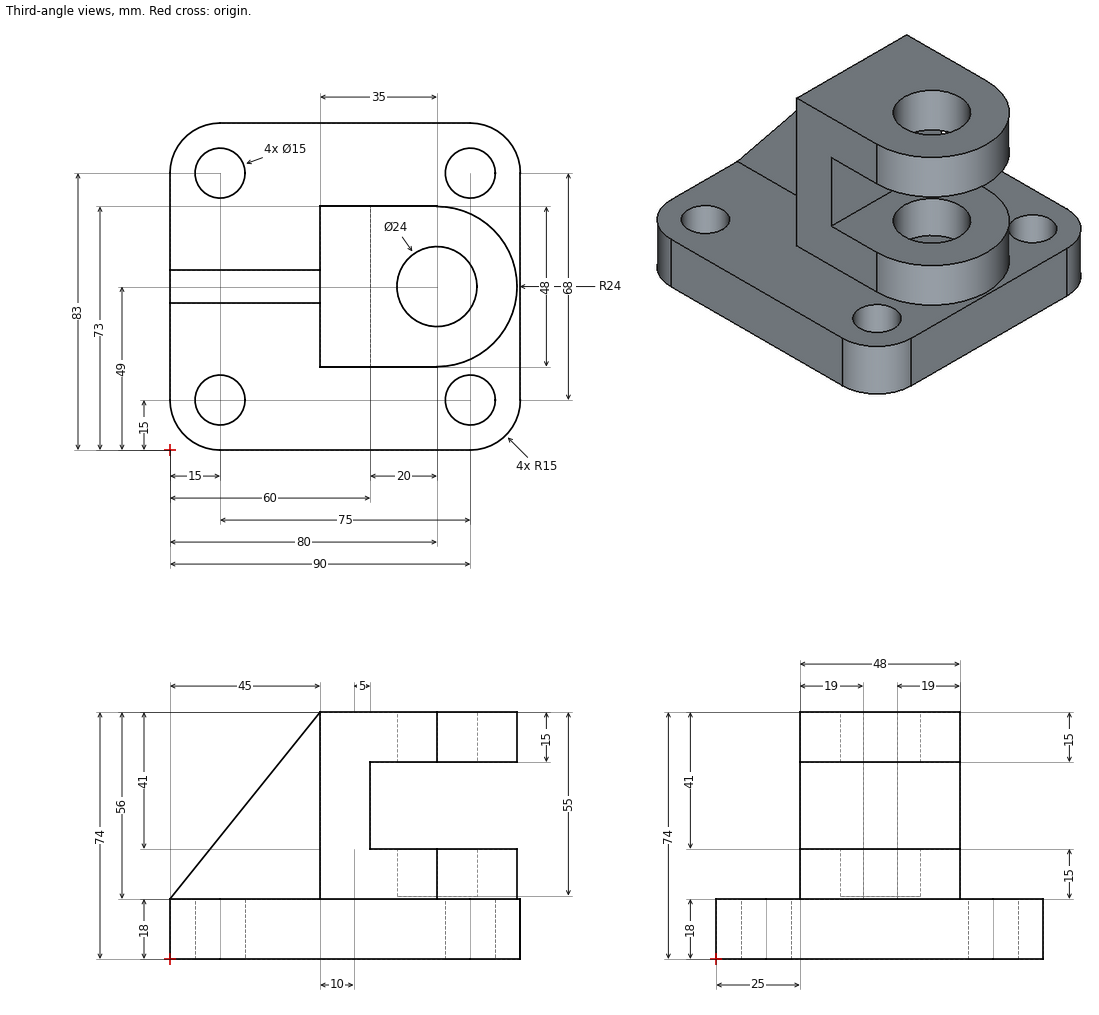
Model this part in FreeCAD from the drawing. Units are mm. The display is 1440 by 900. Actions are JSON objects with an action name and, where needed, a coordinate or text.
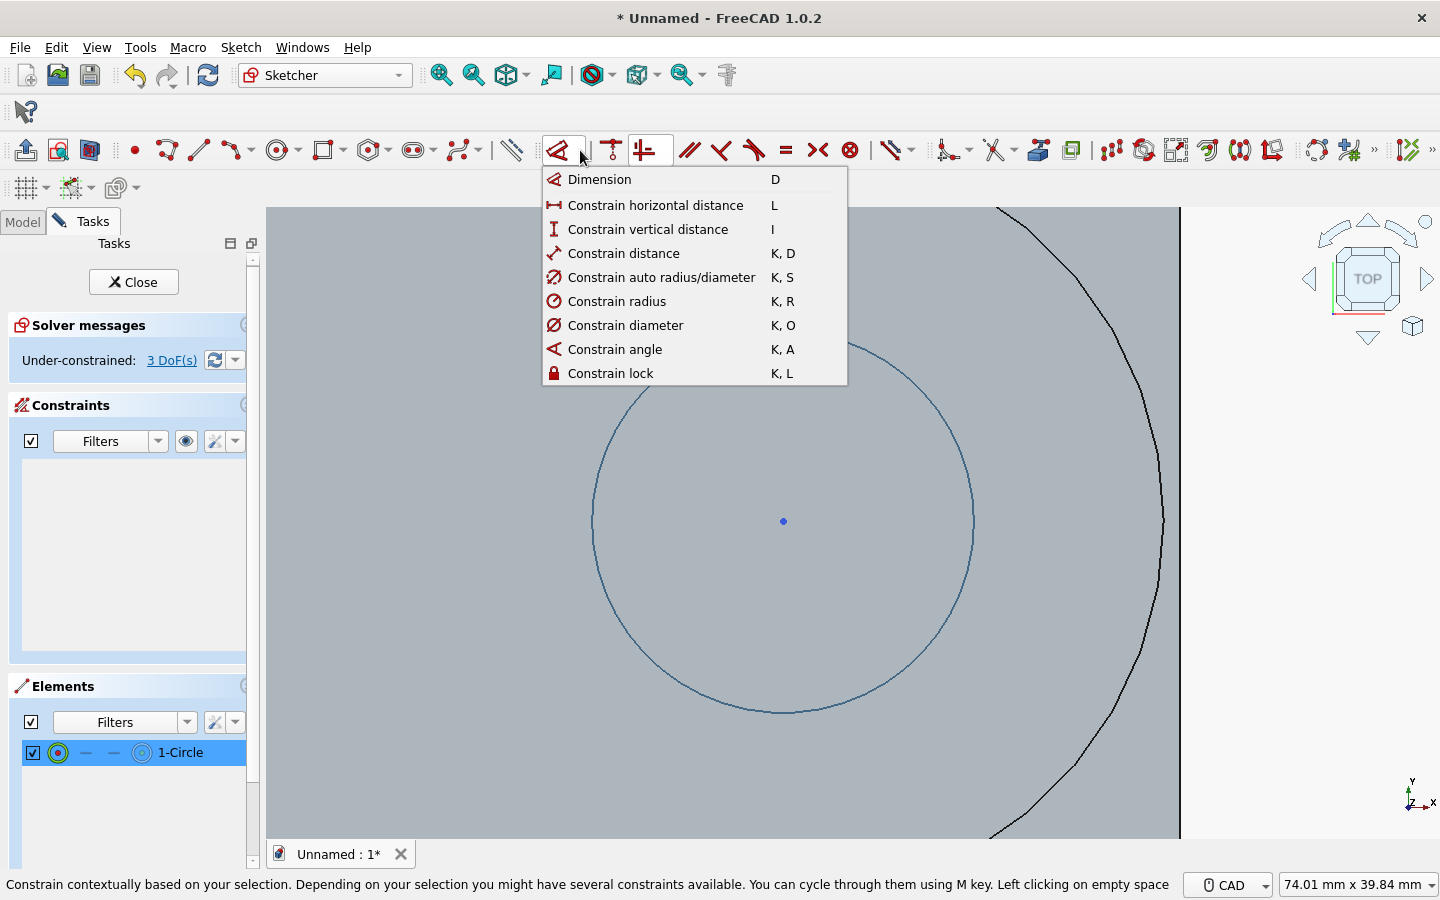
{"action": "left_click", "coordinate": [695, 325]}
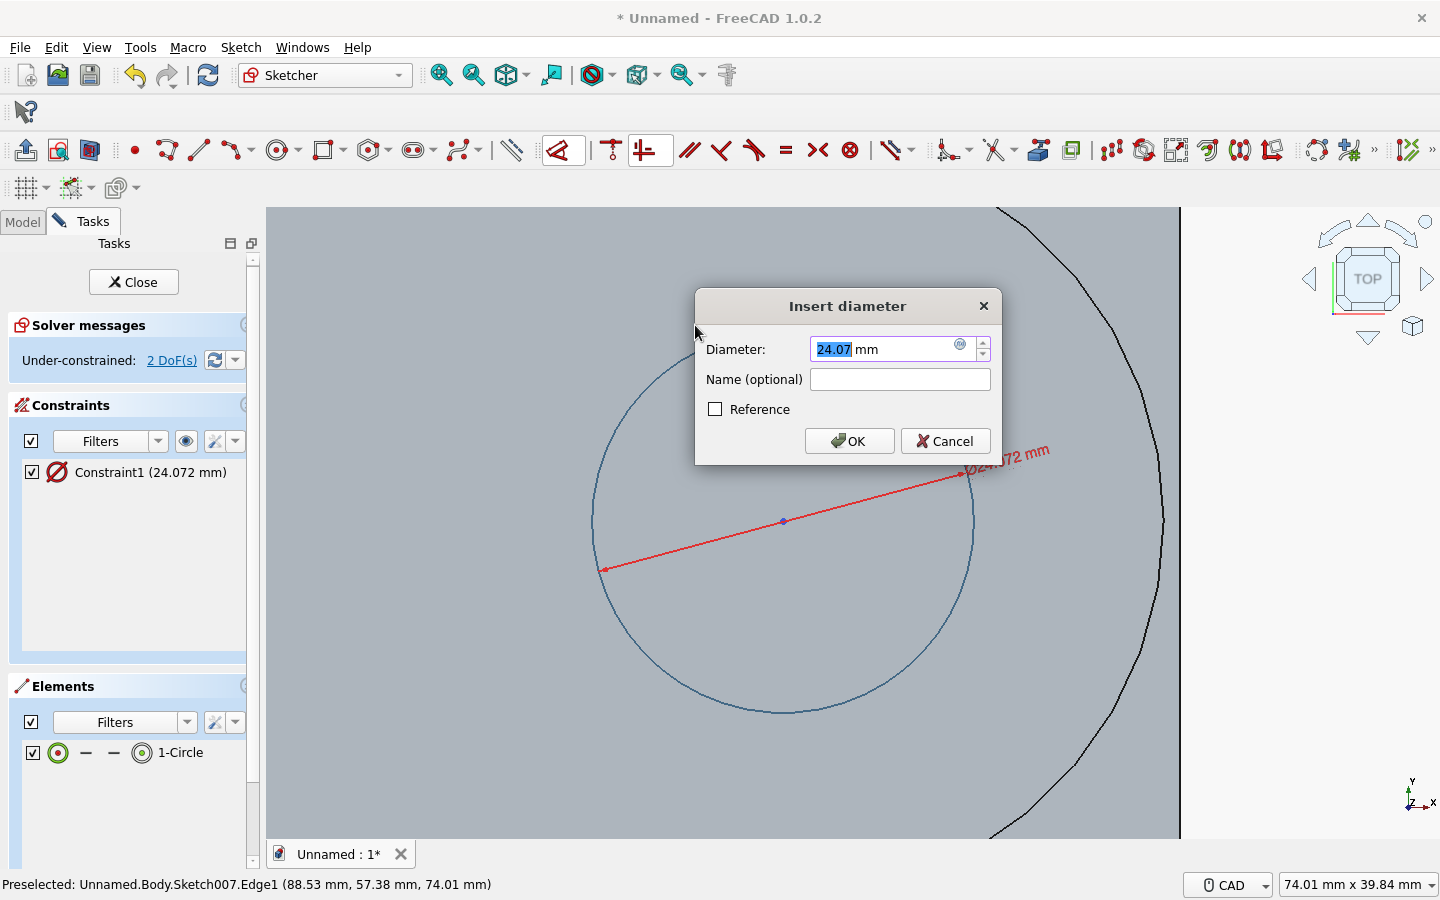
{"action": "type", "text": "24"}
{"action": "key", "text": "Return"}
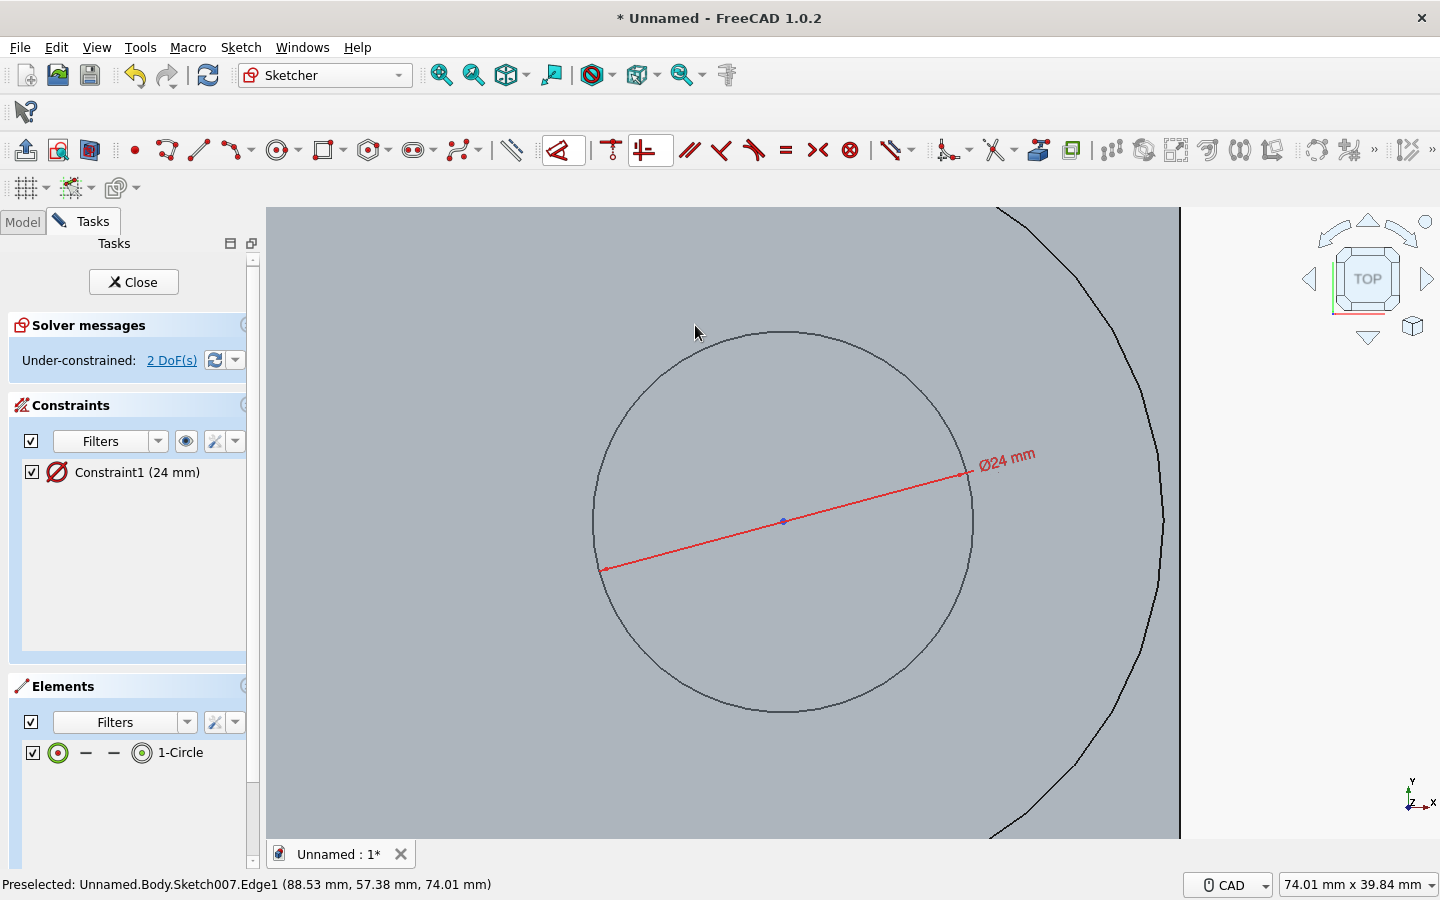
{"action": "left_click", "coordinate": [783, 522]}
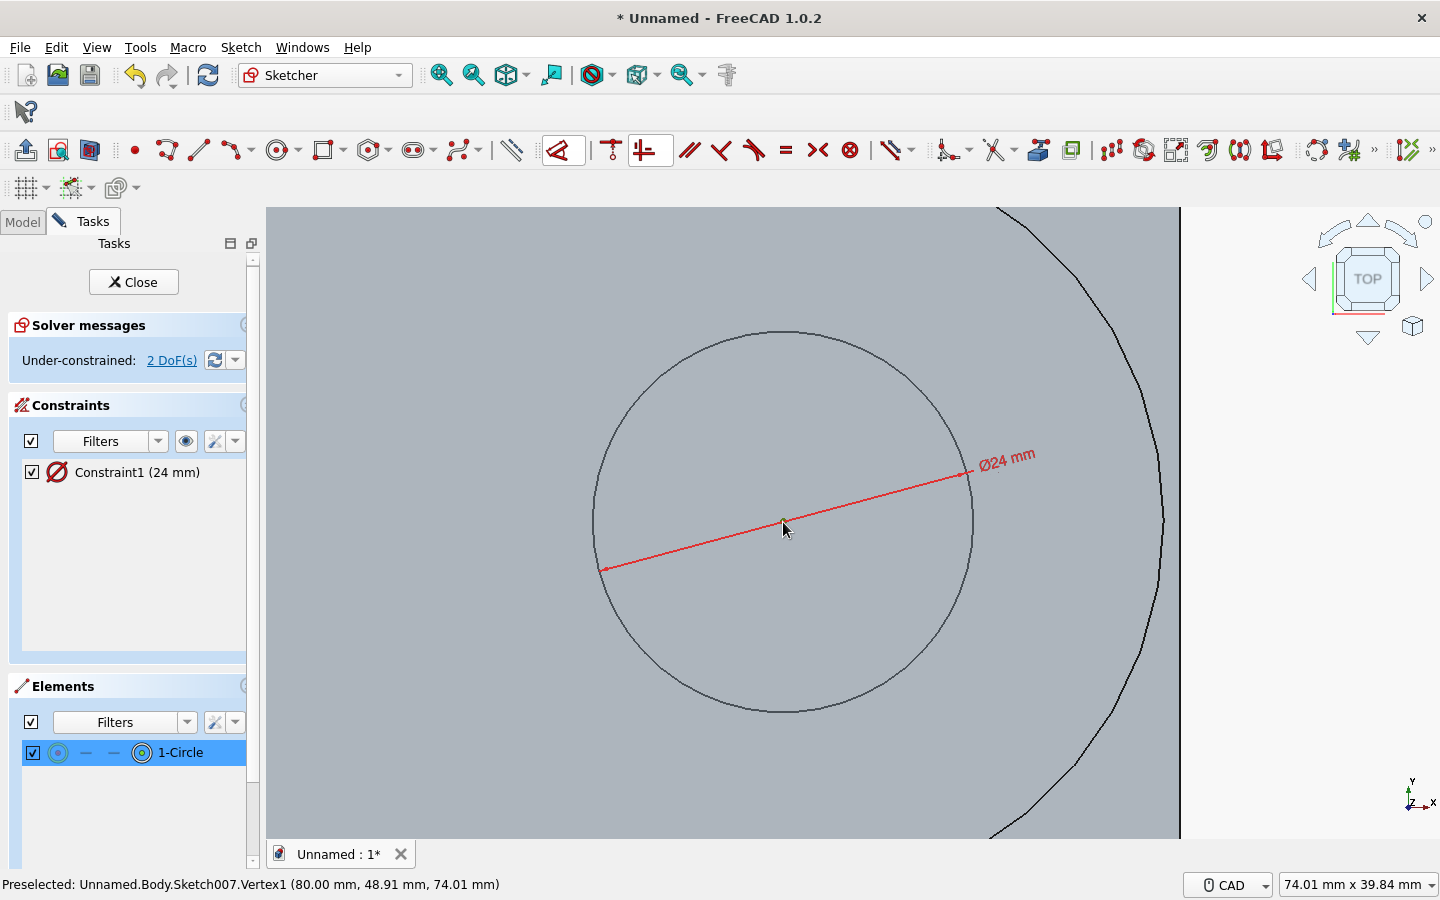
{"action": "left_click", "coordinate": [580, 150]}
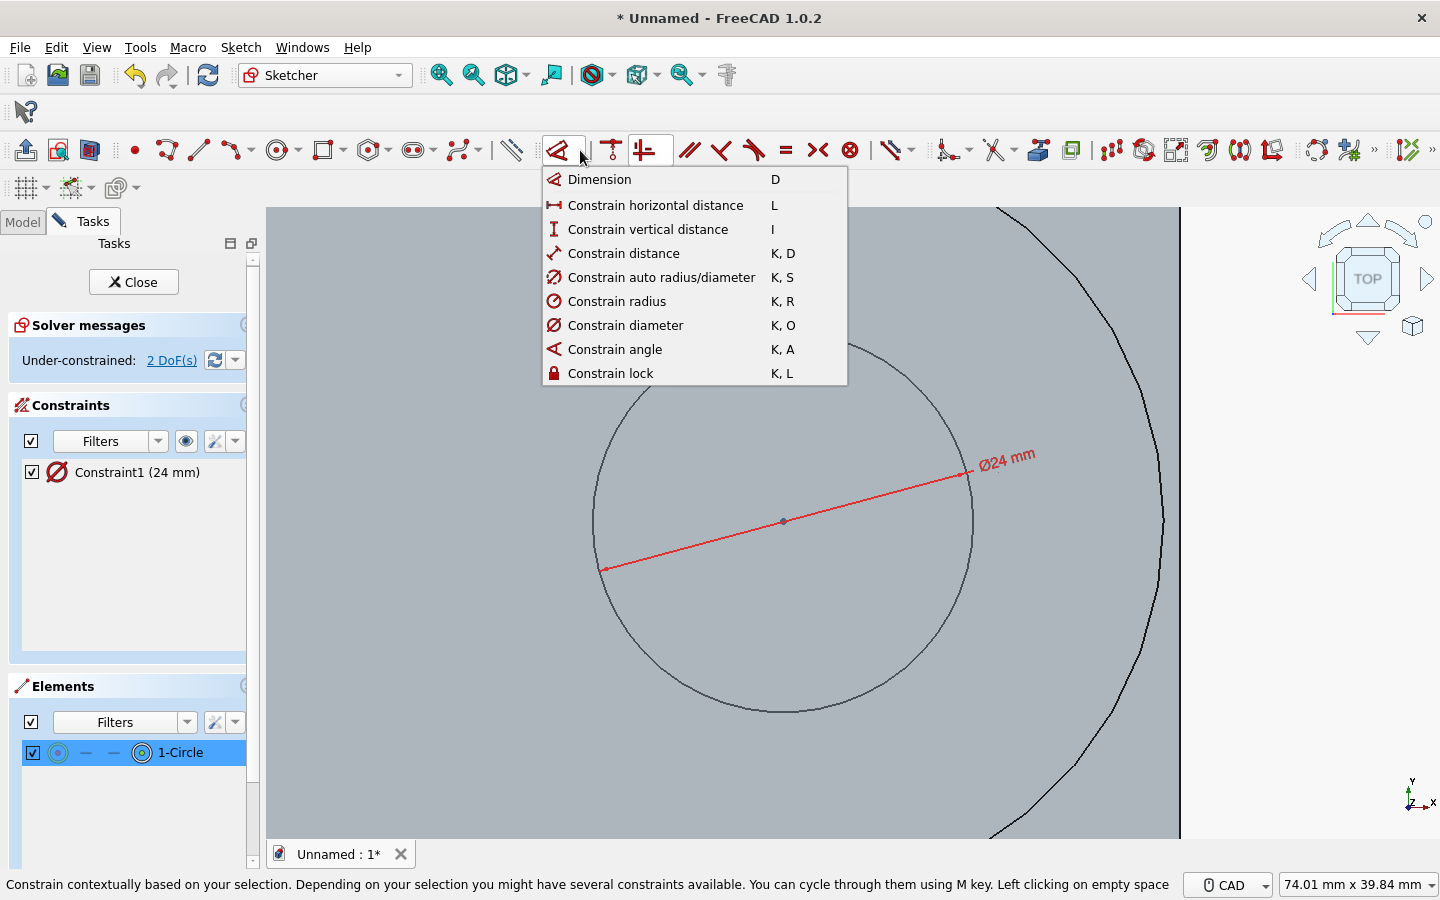
{"action": "left_click", "coordinate": [695, 205]}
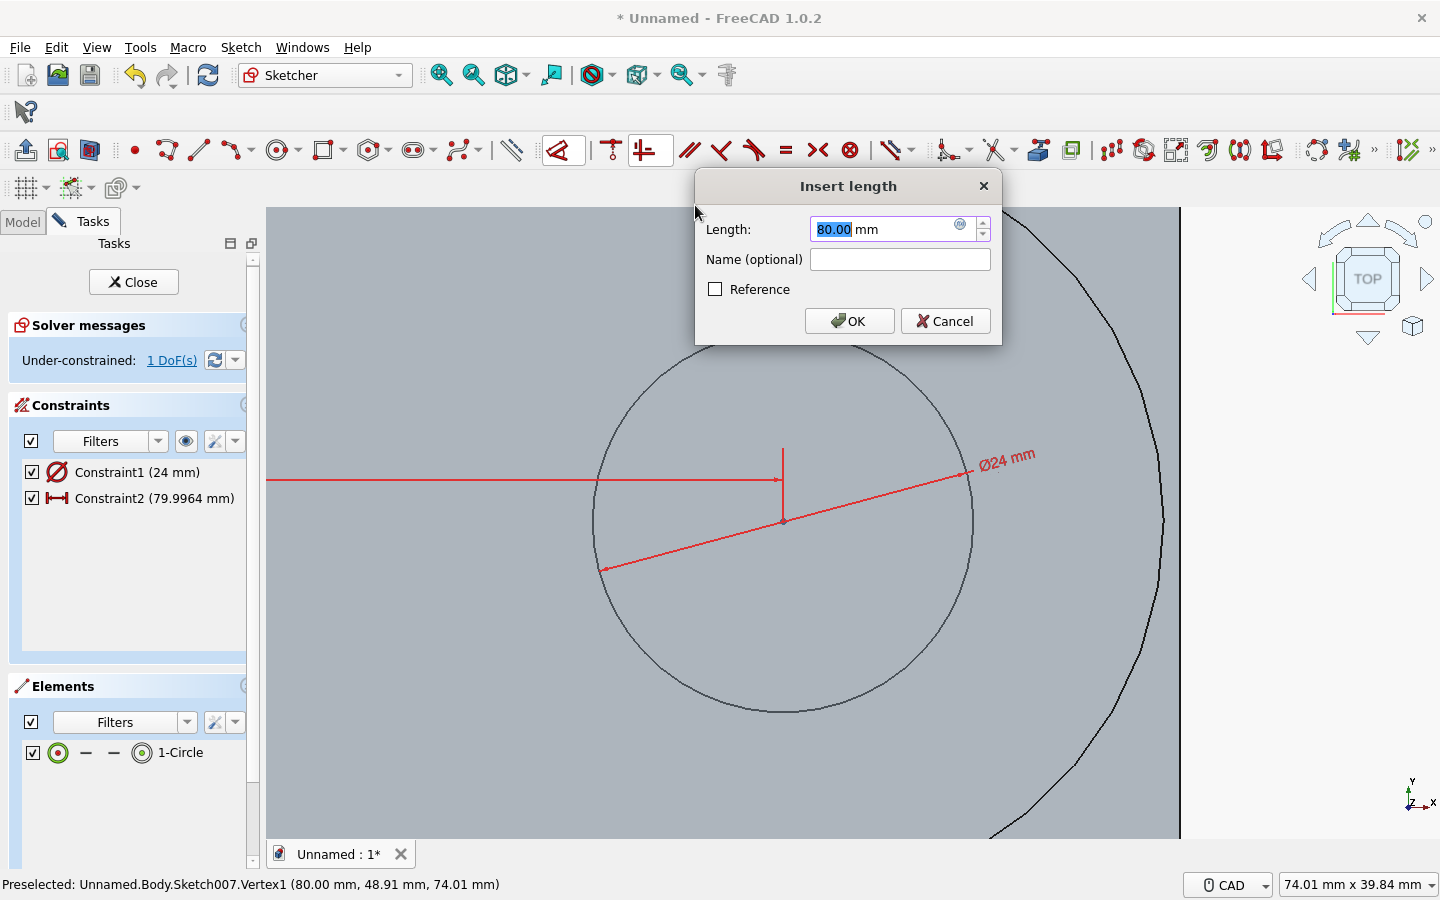
{"action": "type", "text": "80"}
{"action": "key", "text": "Return"}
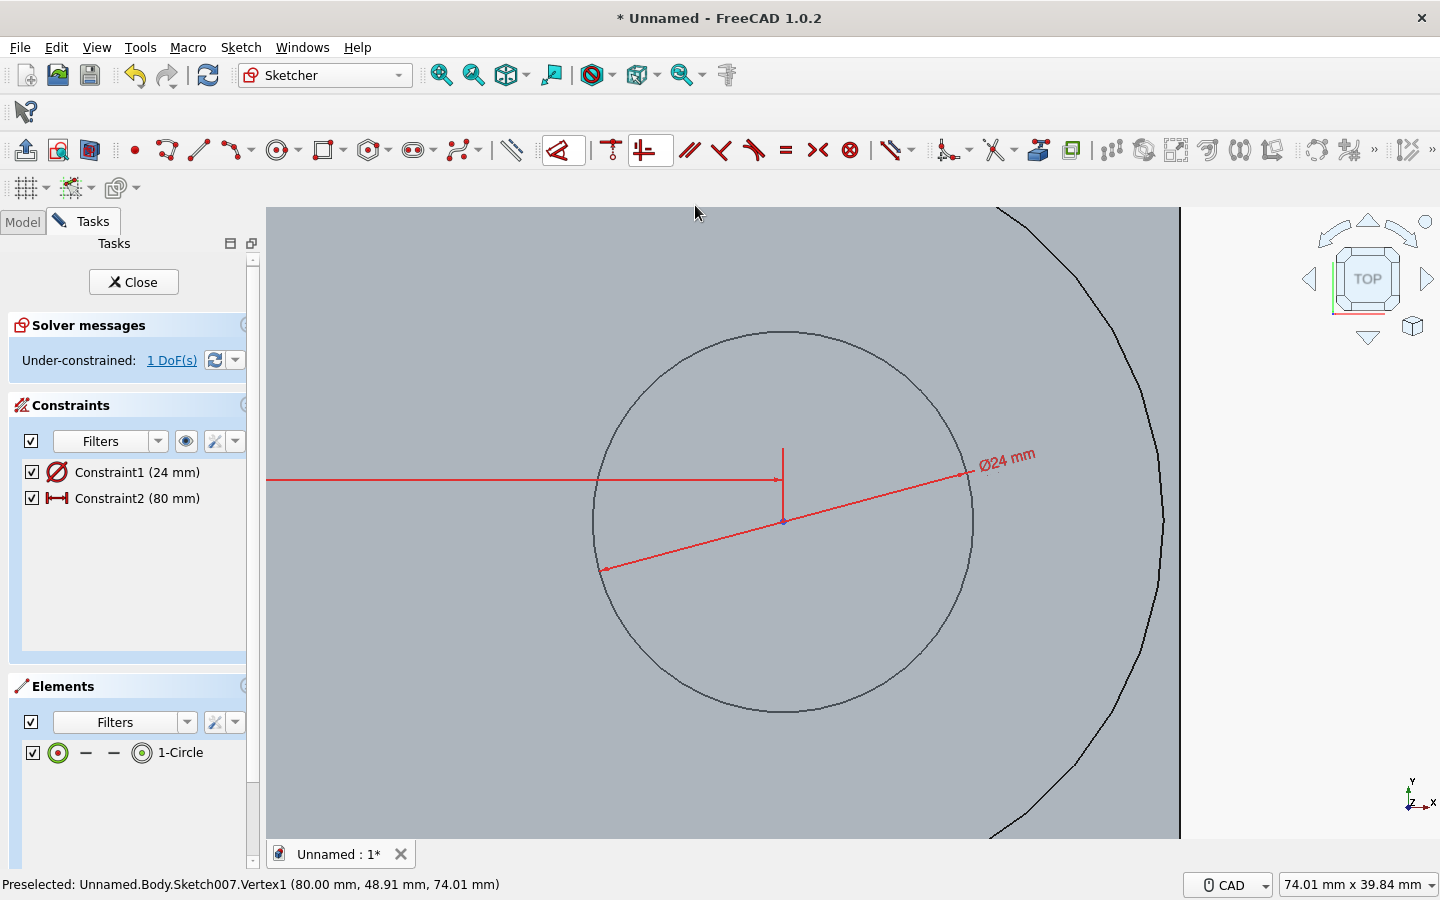
{"action": "left_click", "coordinate": [783, 522]}